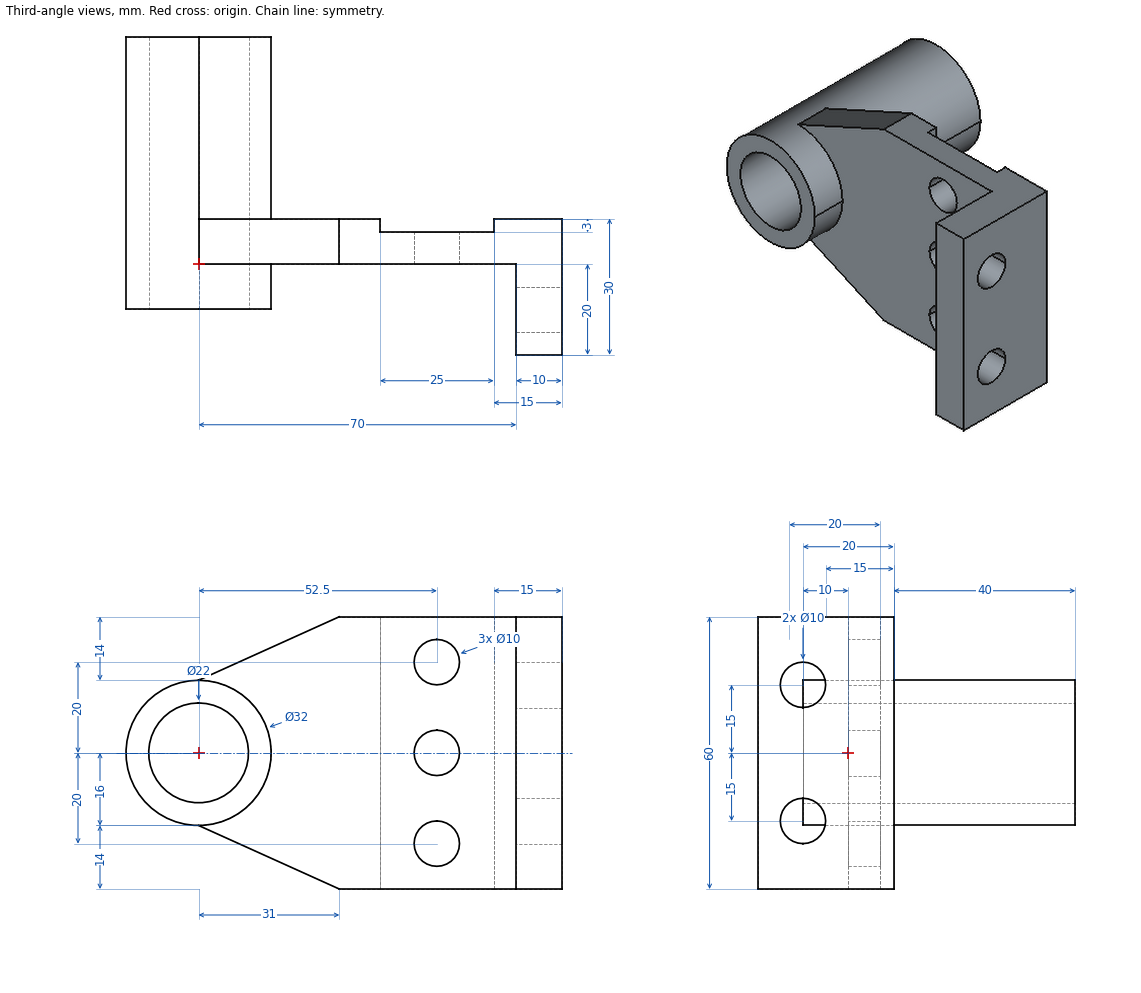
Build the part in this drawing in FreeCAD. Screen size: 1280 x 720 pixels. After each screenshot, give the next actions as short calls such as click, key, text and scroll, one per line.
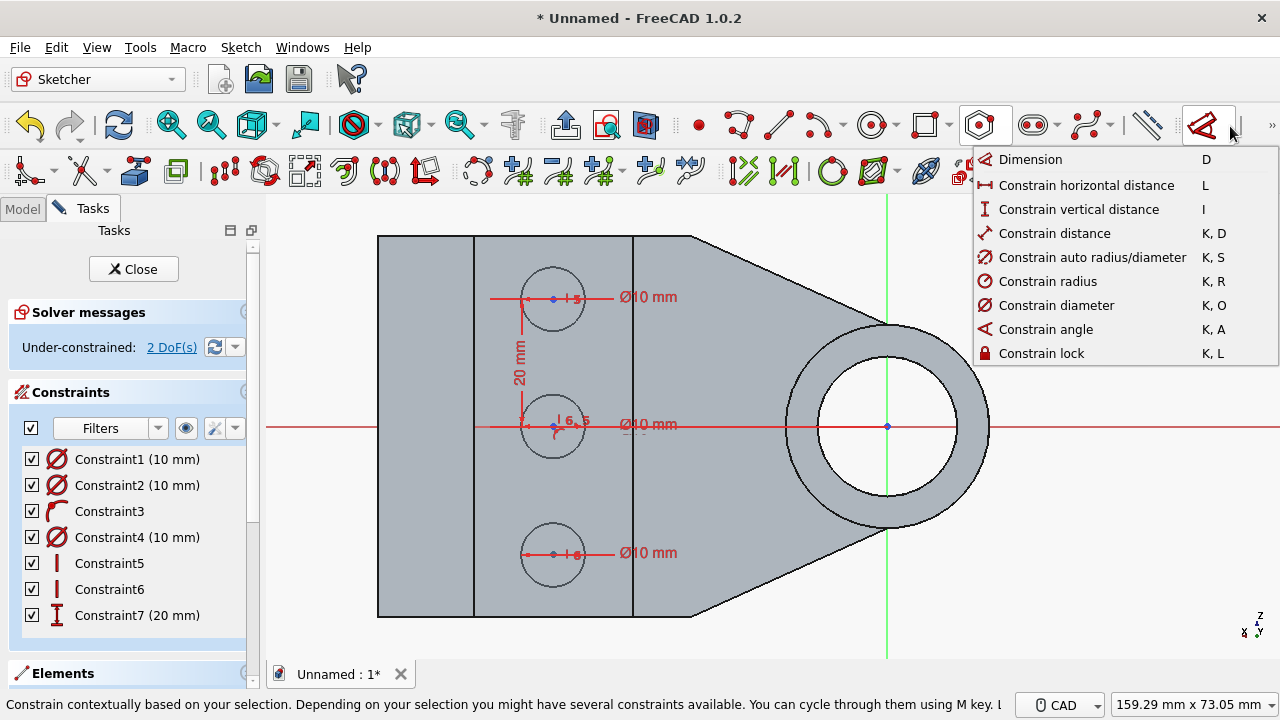
click(1126, 209)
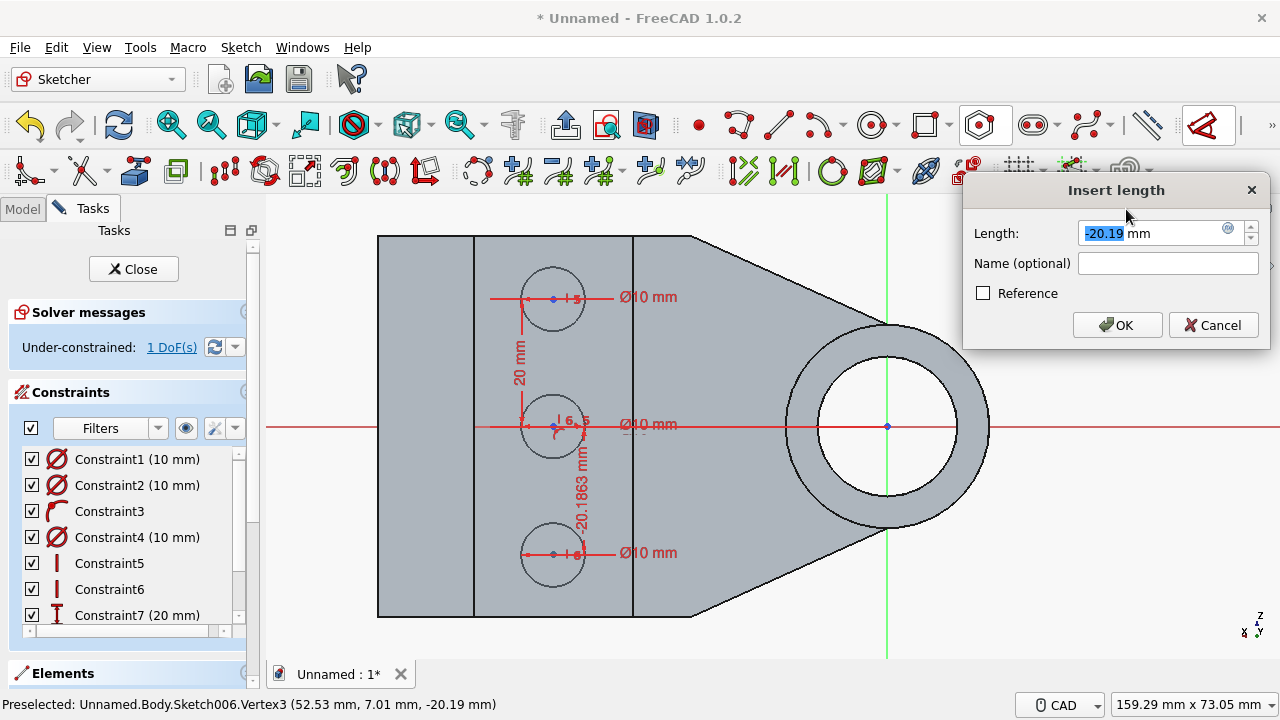
text(-20)
key(Return)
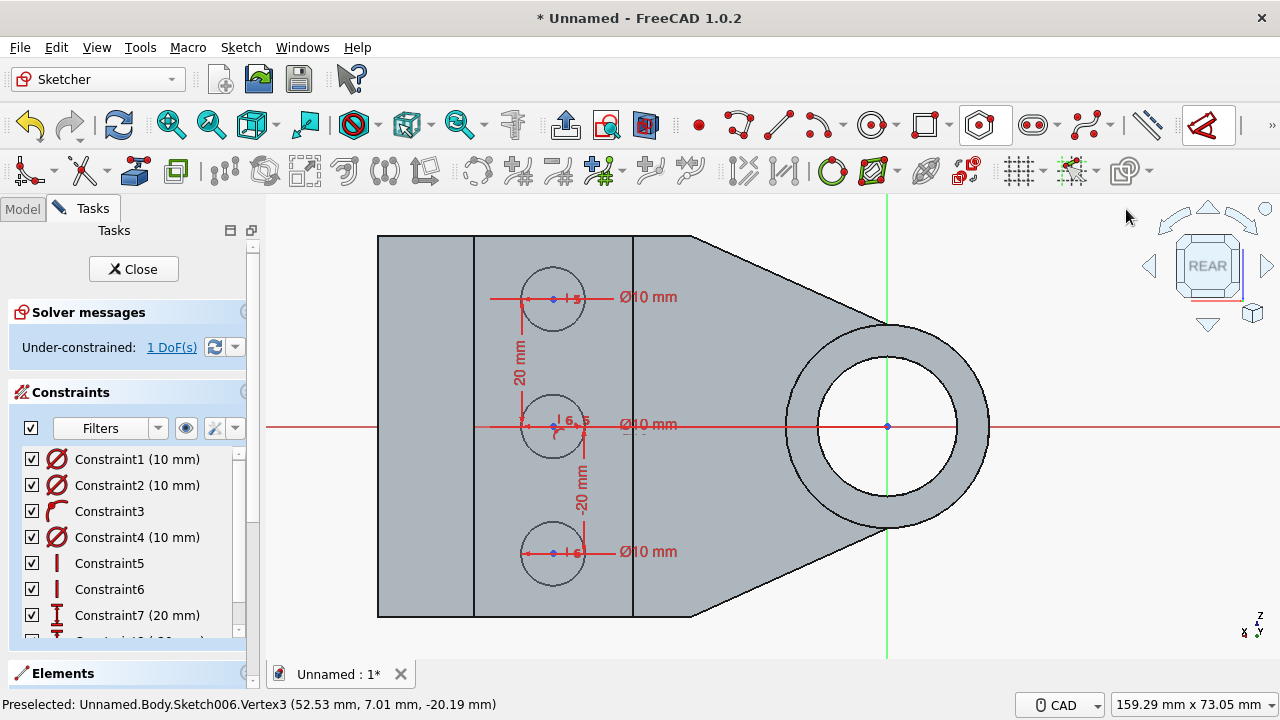
click(553, 299)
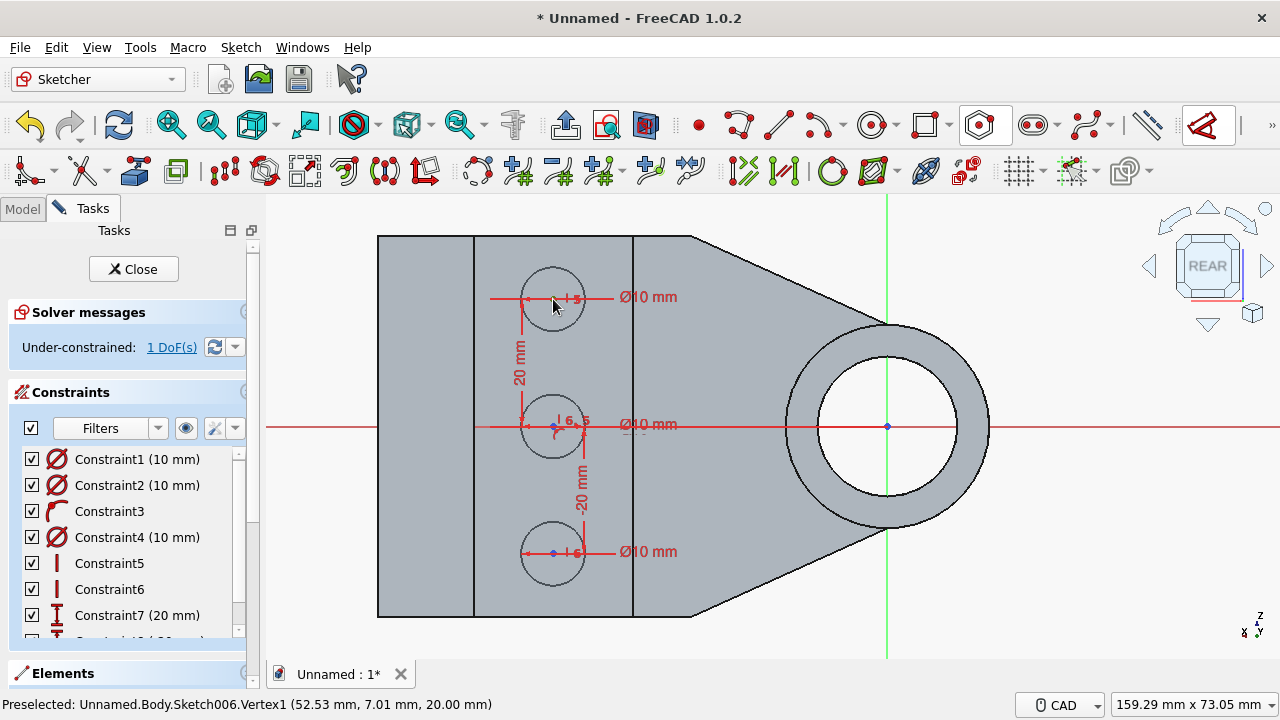
key(l)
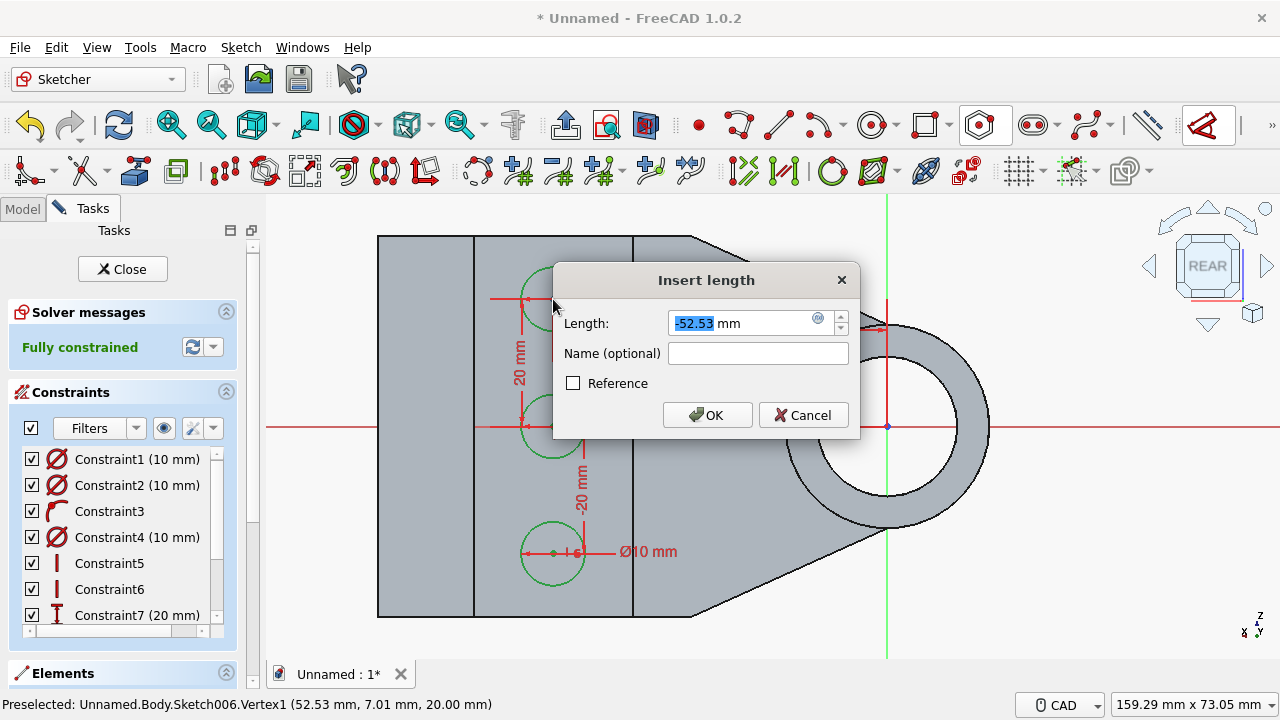
text(-52.5)
key(Return)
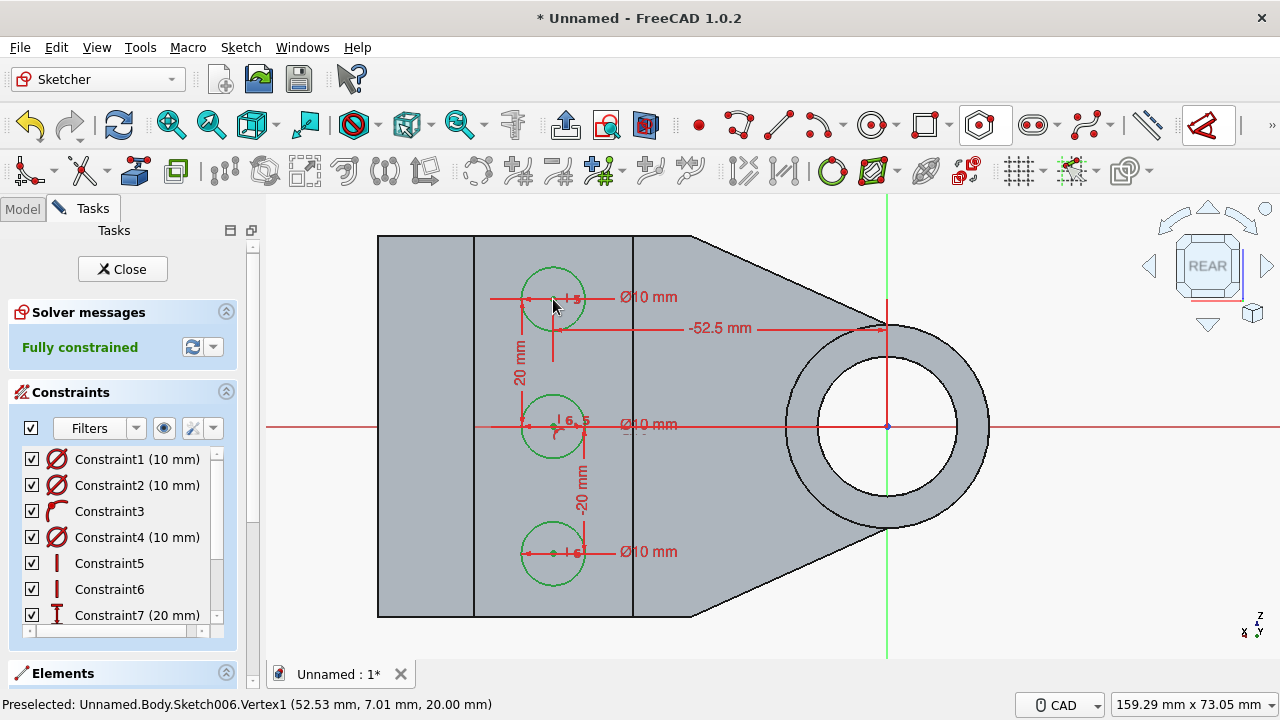
click(123, 269)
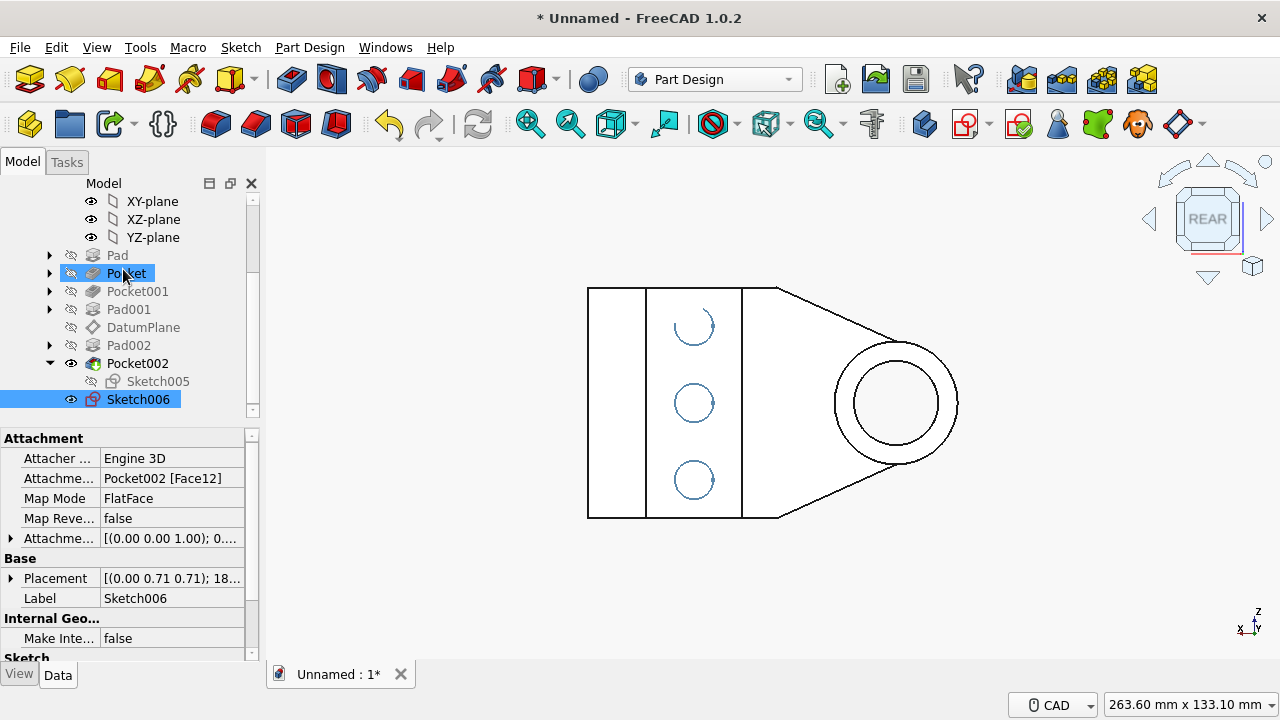
click(292, 80)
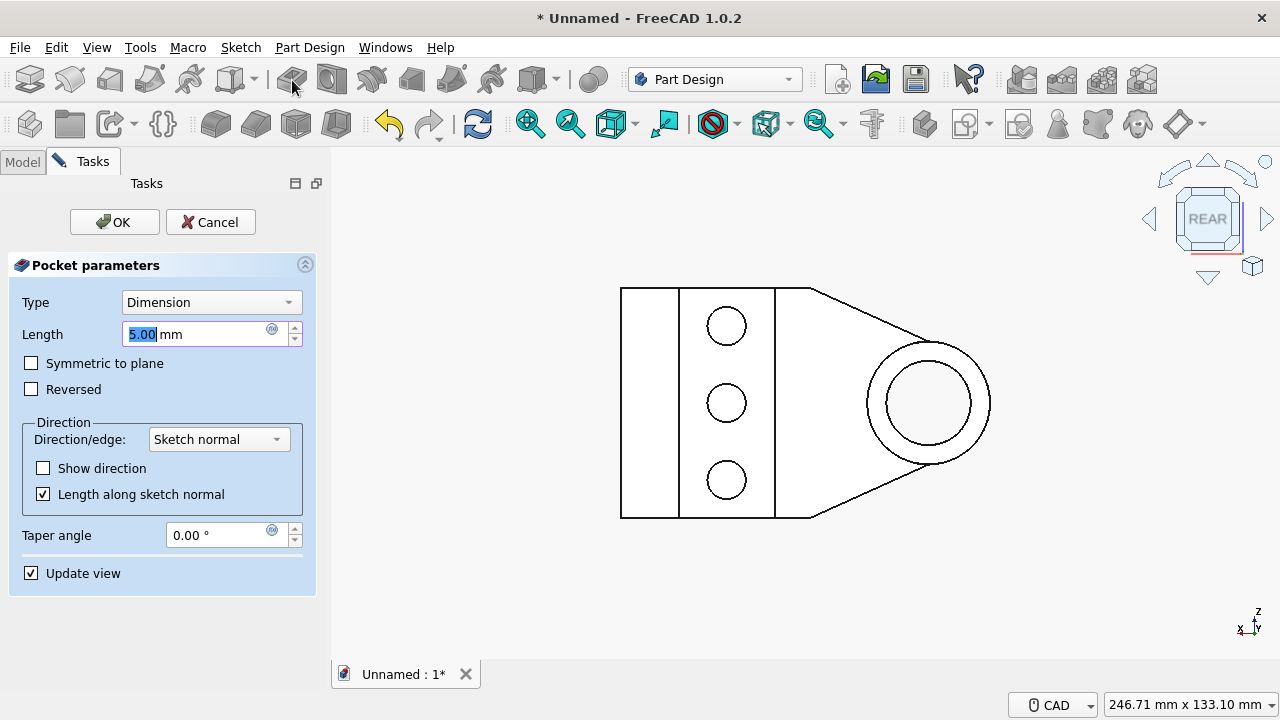
text(20)
key(Tab)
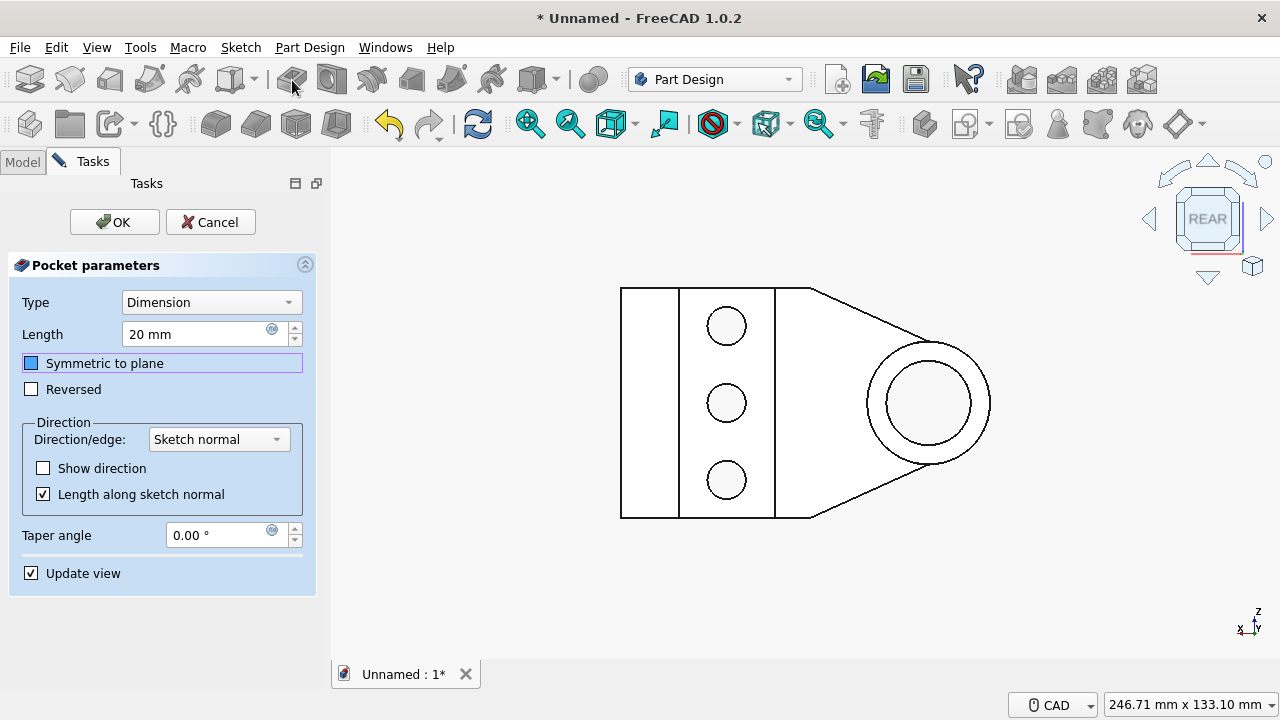
click(115, 222)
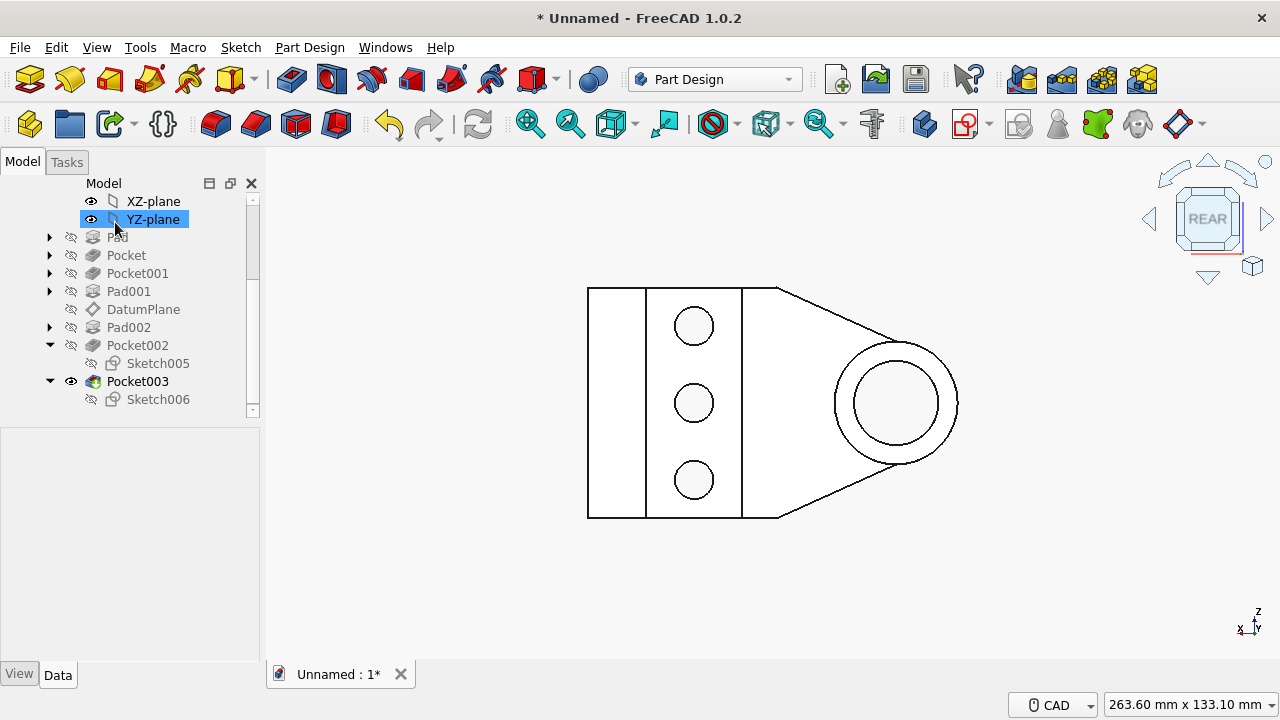
key(0)